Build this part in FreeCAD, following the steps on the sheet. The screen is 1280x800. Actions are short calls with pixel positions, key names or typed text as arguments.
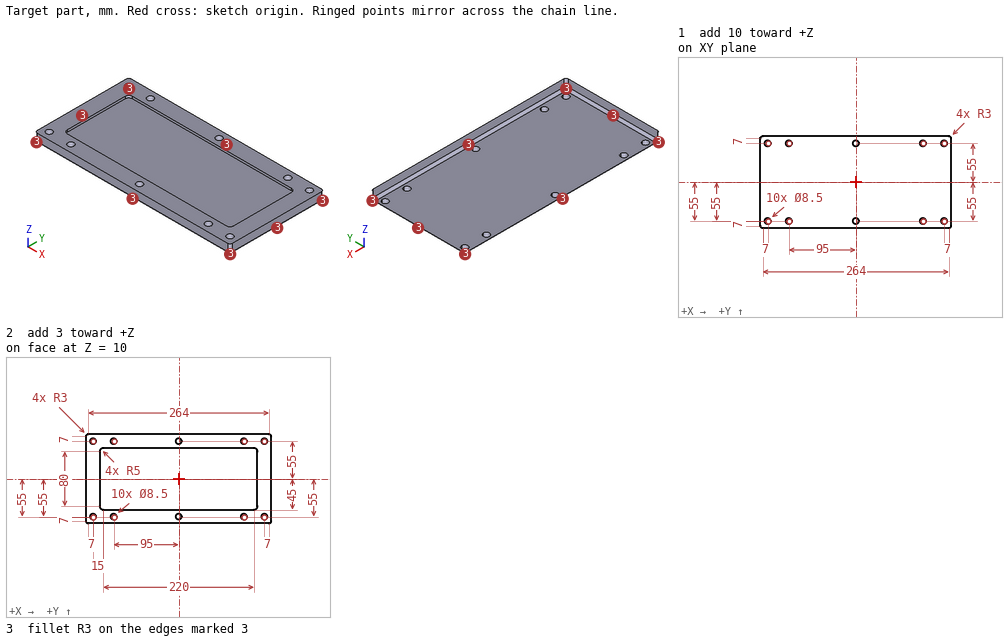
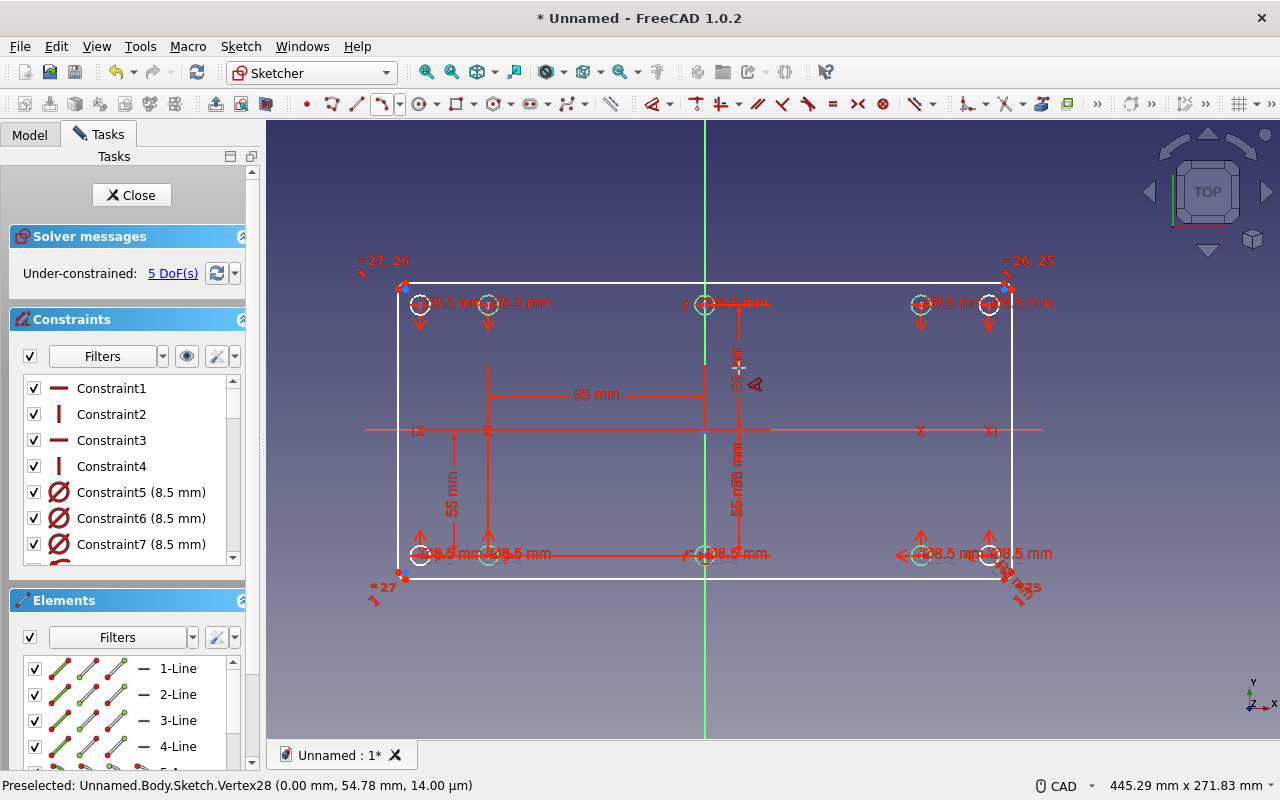
scroll(405, 579, up, 5)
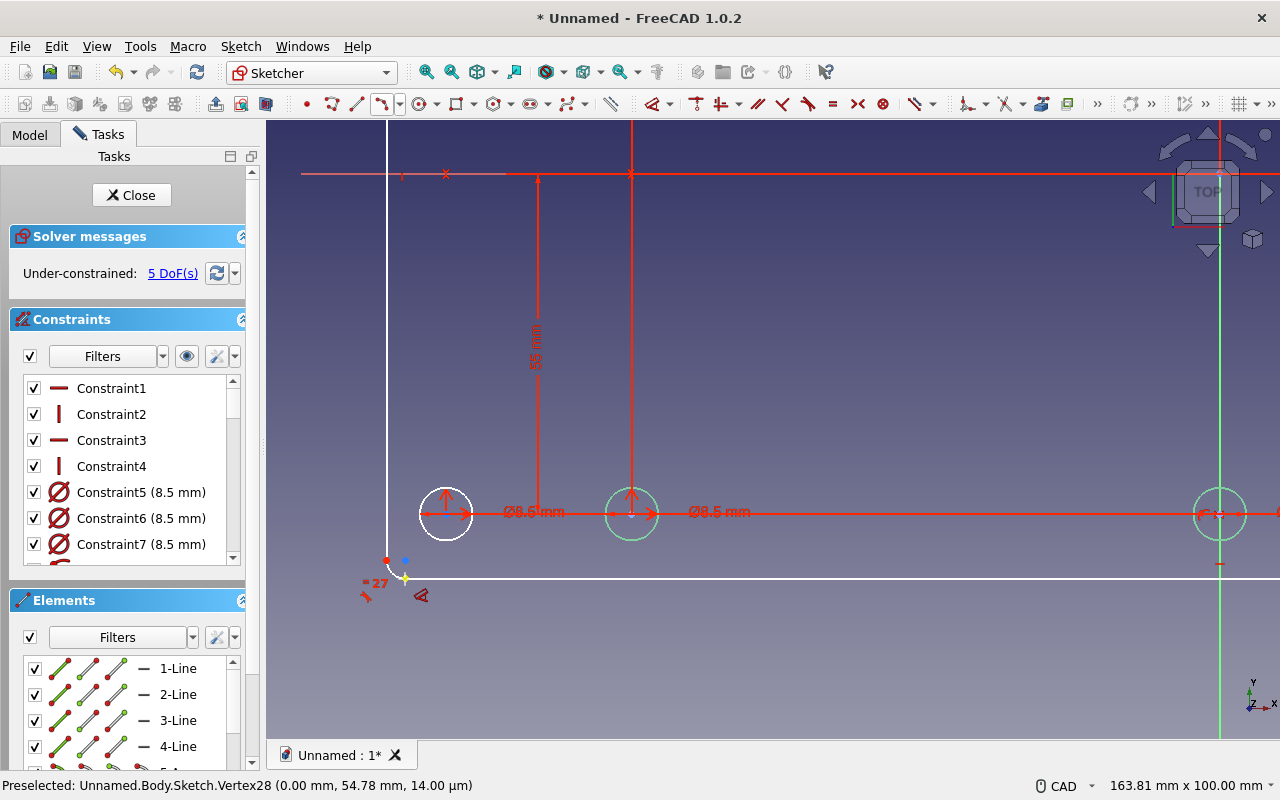
click(405, 579)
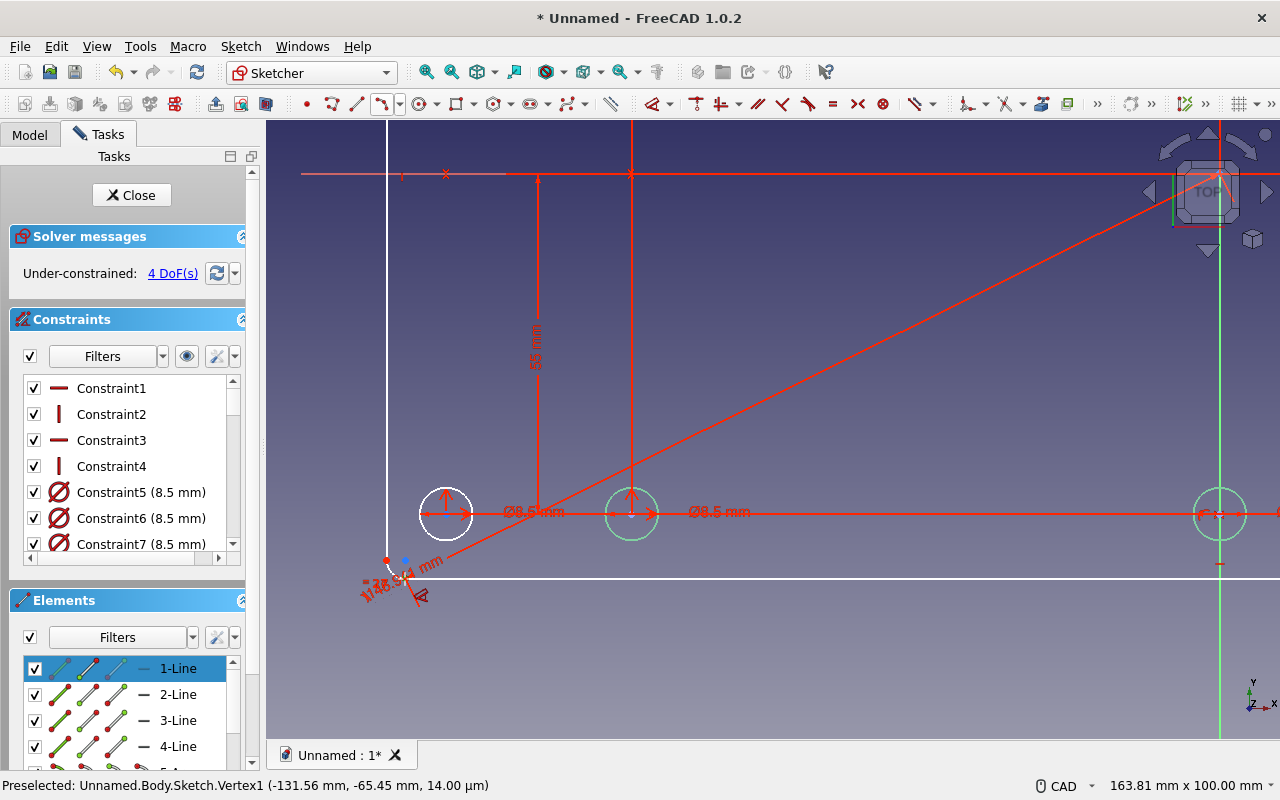
click(446, 514)
click(426, 613)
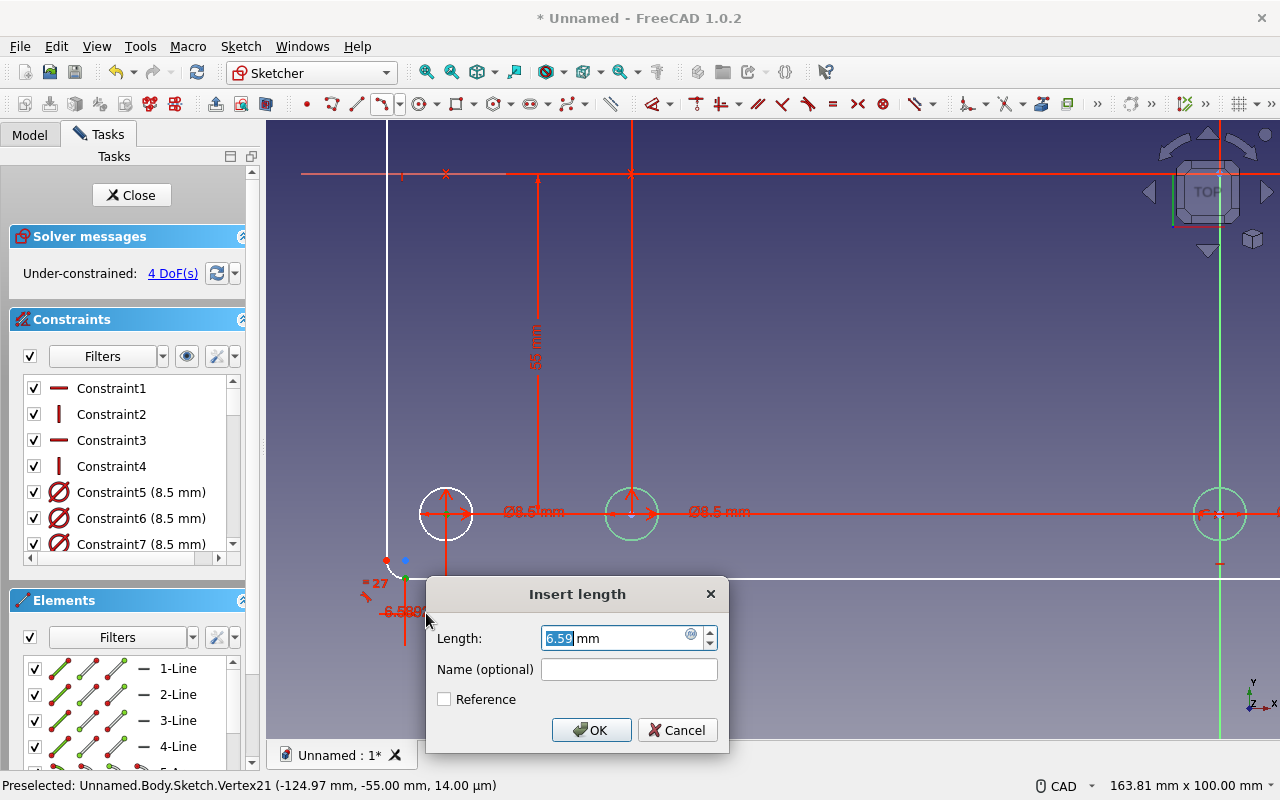
text(7)
key(Return)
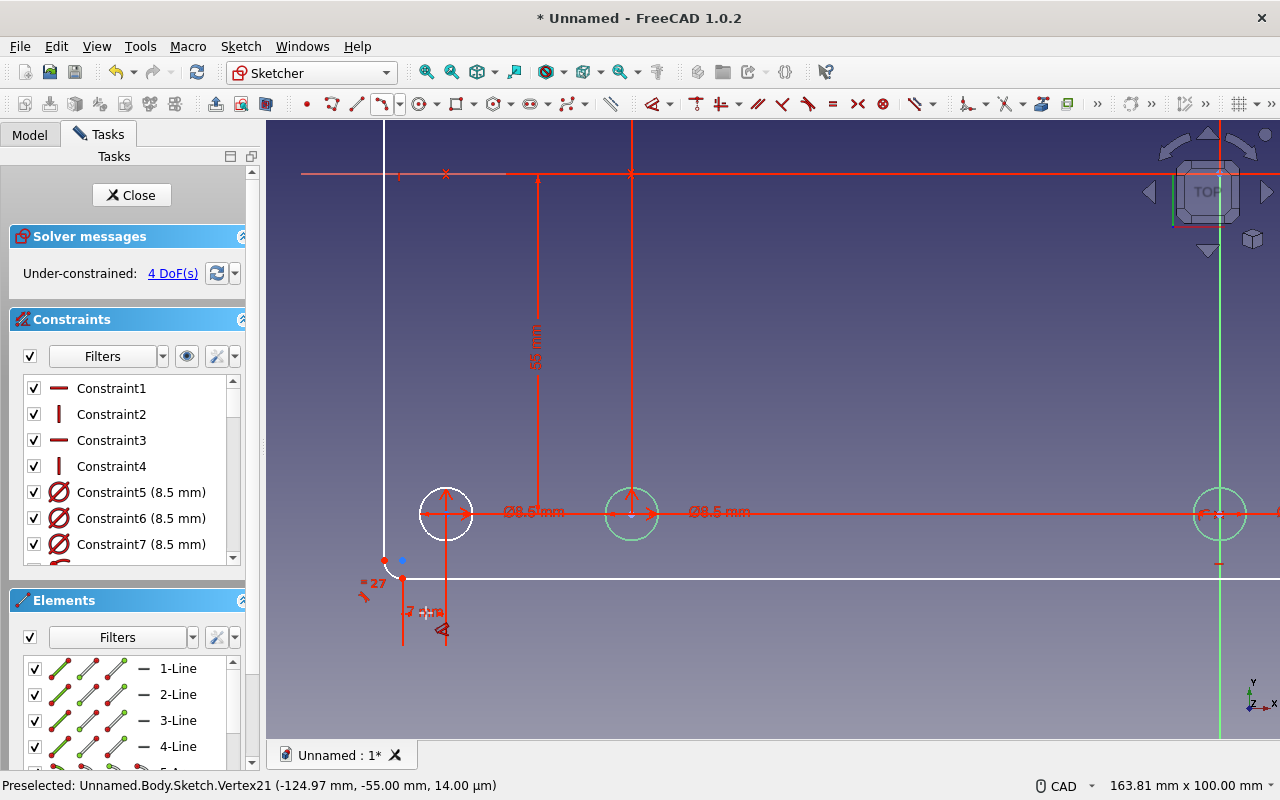
click(384, 560)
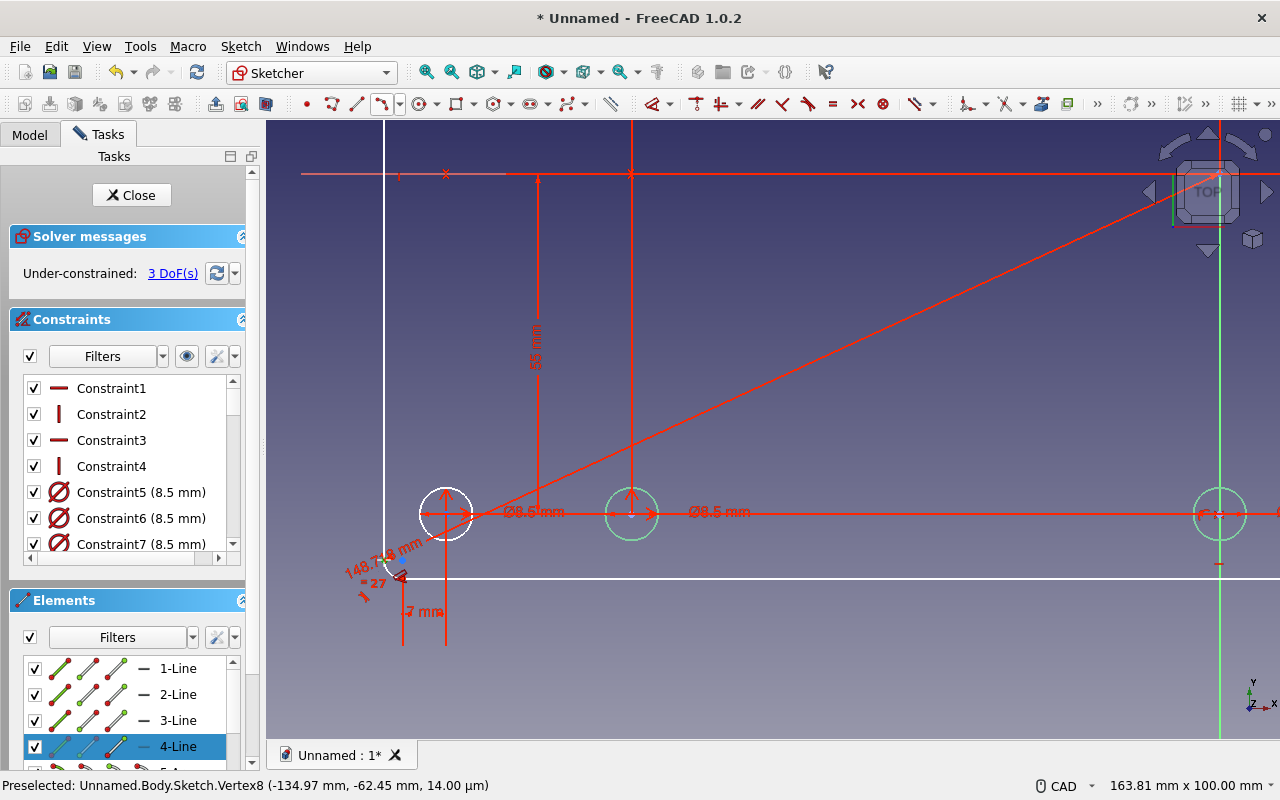
click(446, 514)
click(350, 537)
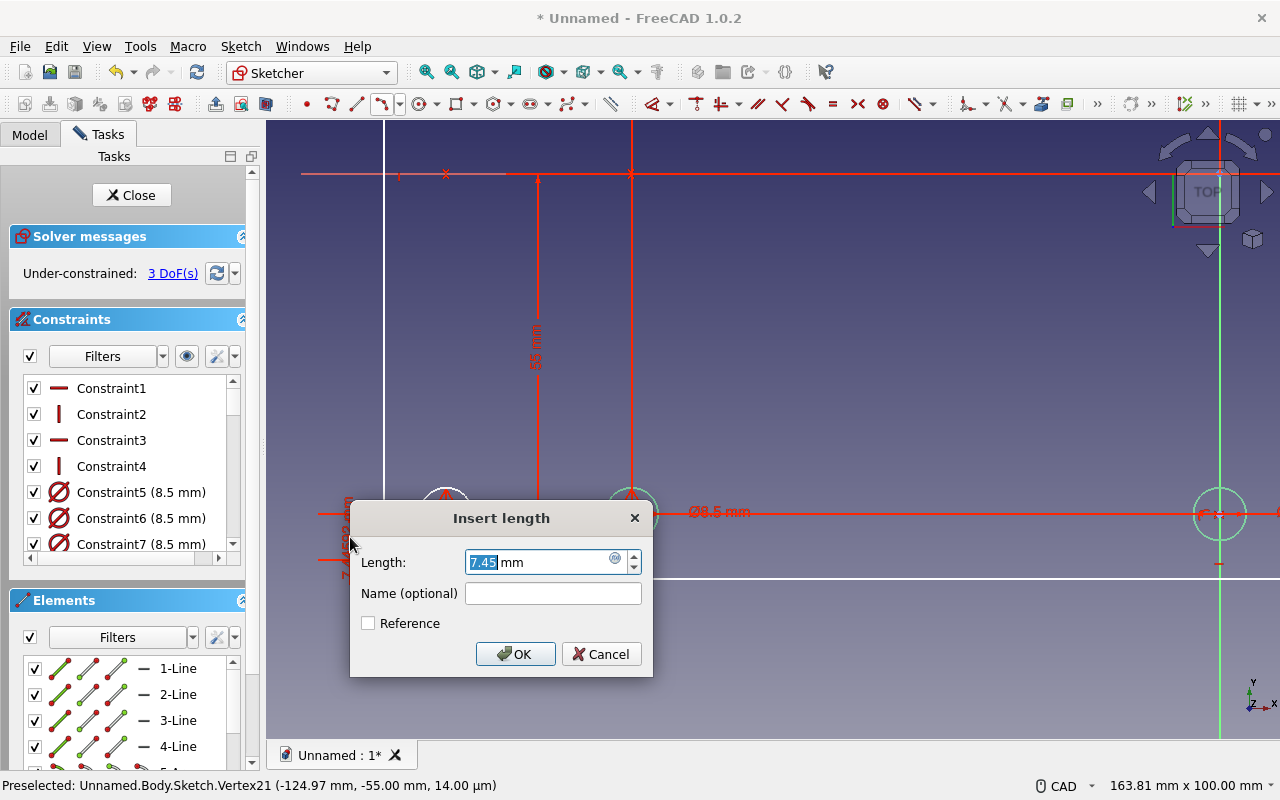
text(7)
key(Return)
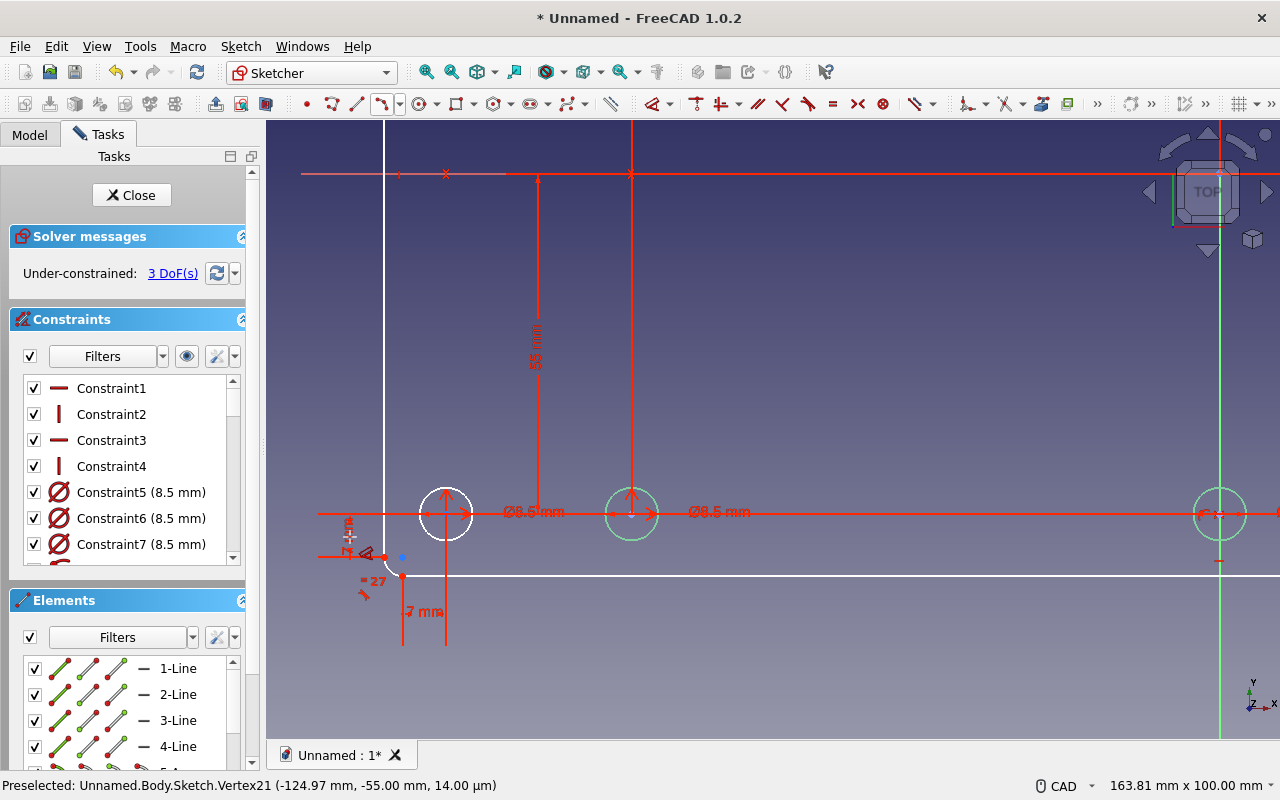
scroll(405, 578, down, 5)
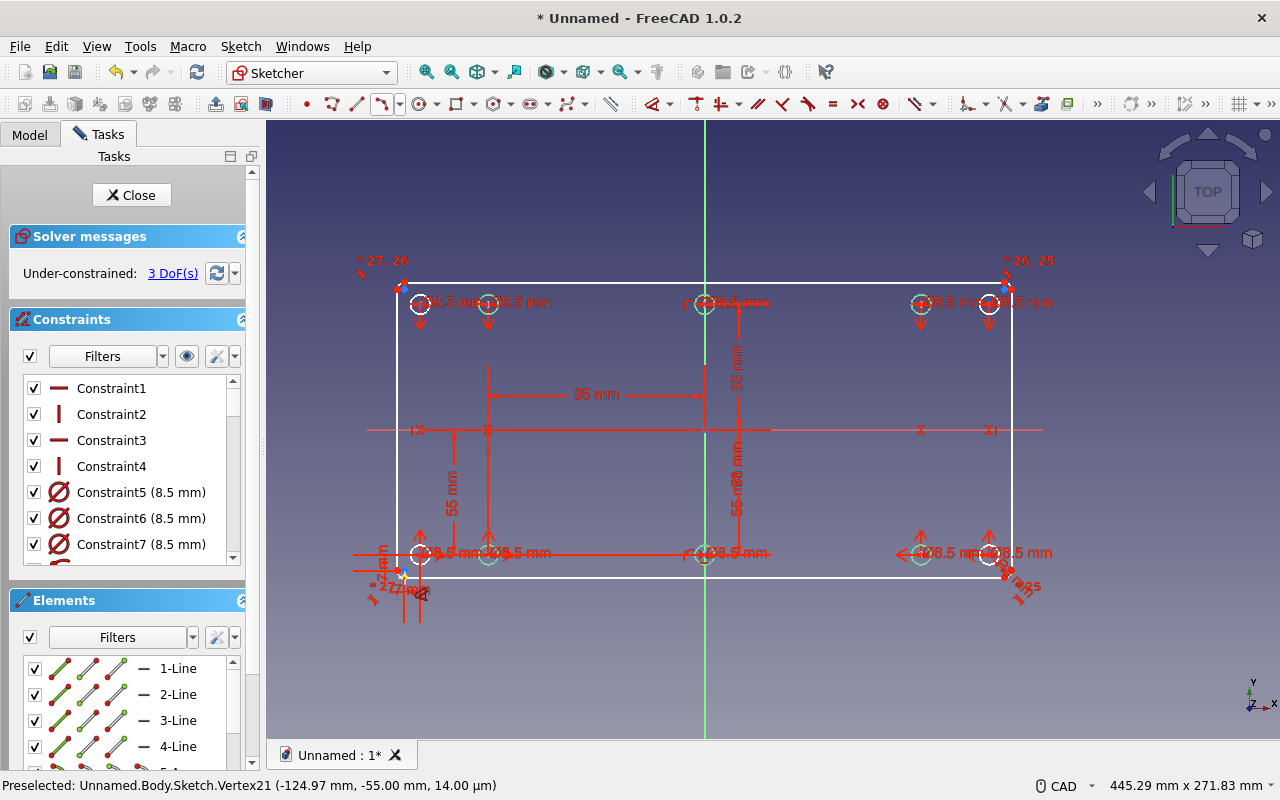
scroll(1005, 578, up, 5)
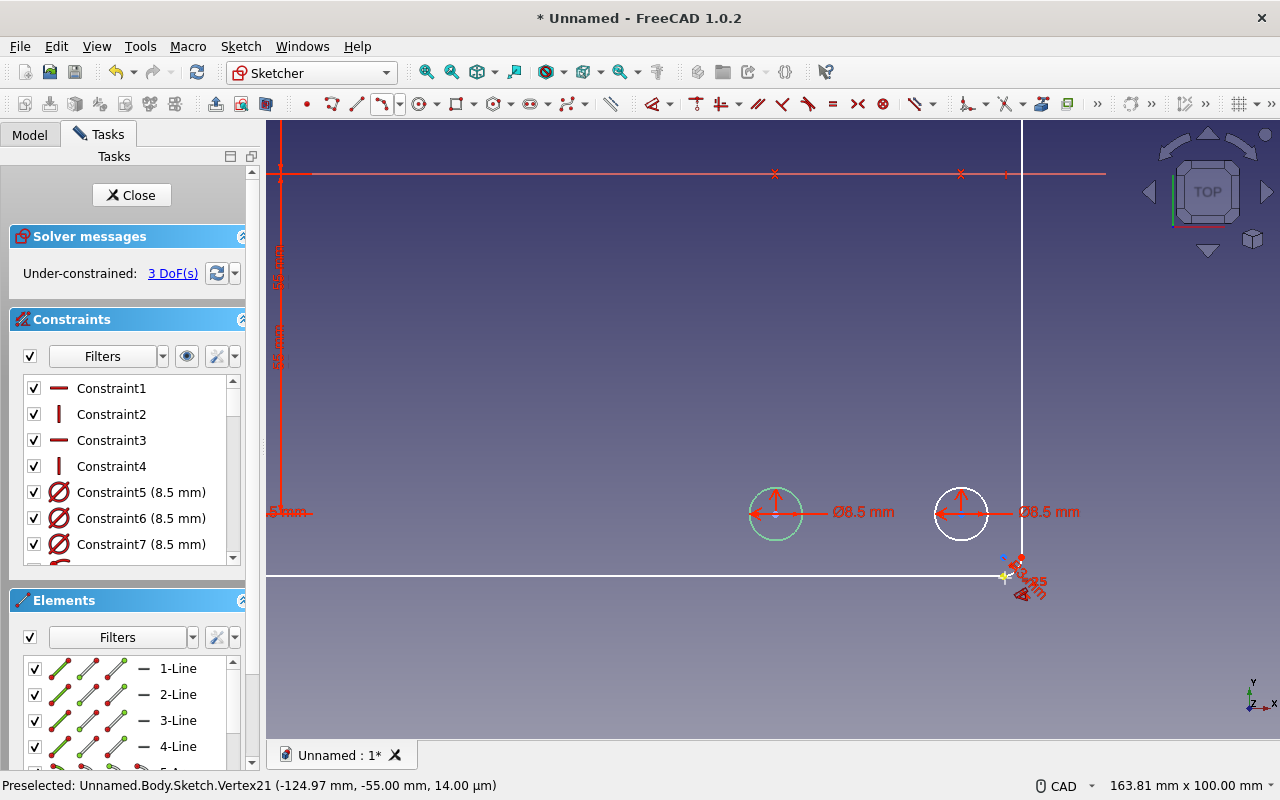
click(1003, 576)